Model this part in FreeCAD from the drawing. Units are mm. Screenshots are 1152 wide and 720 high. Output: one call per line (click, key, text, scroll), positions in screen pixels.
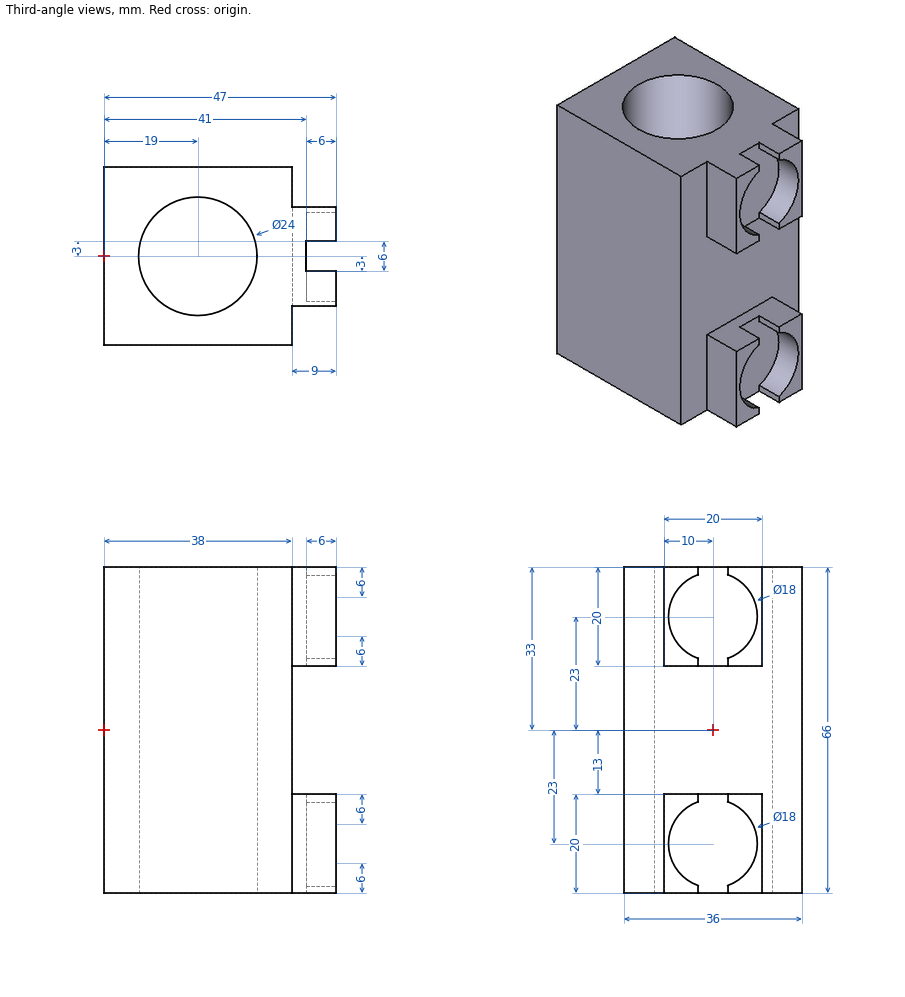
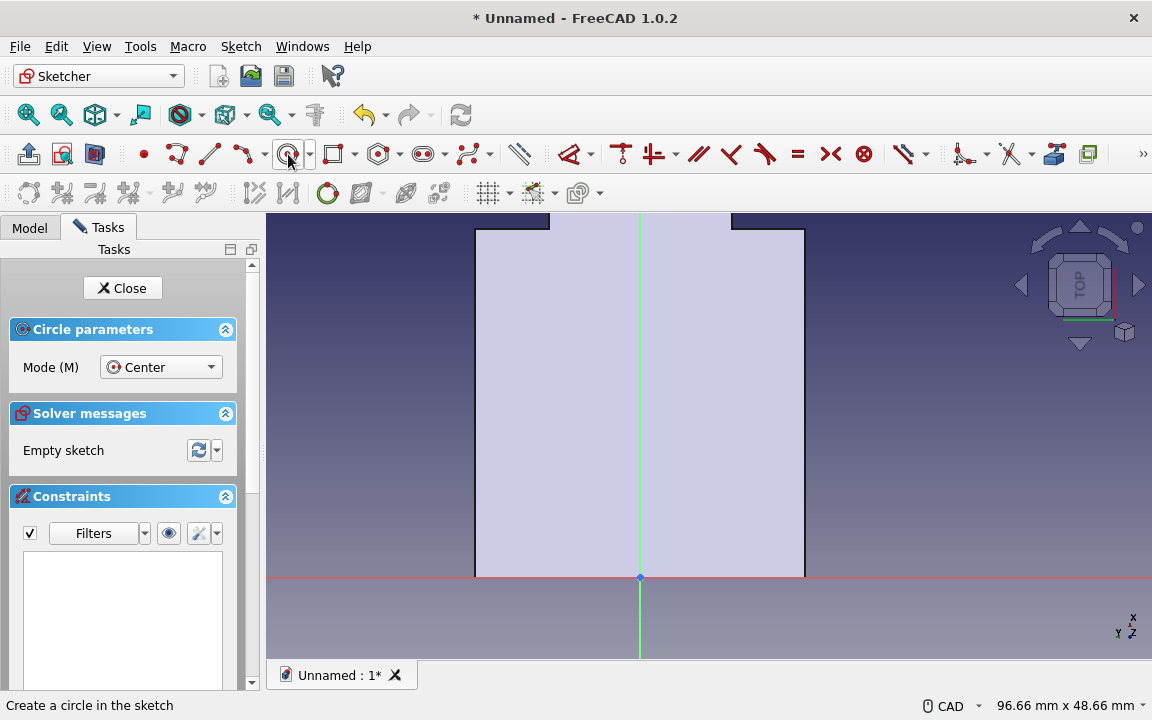
click(640, 404)
click(718, 326)
key(Escape)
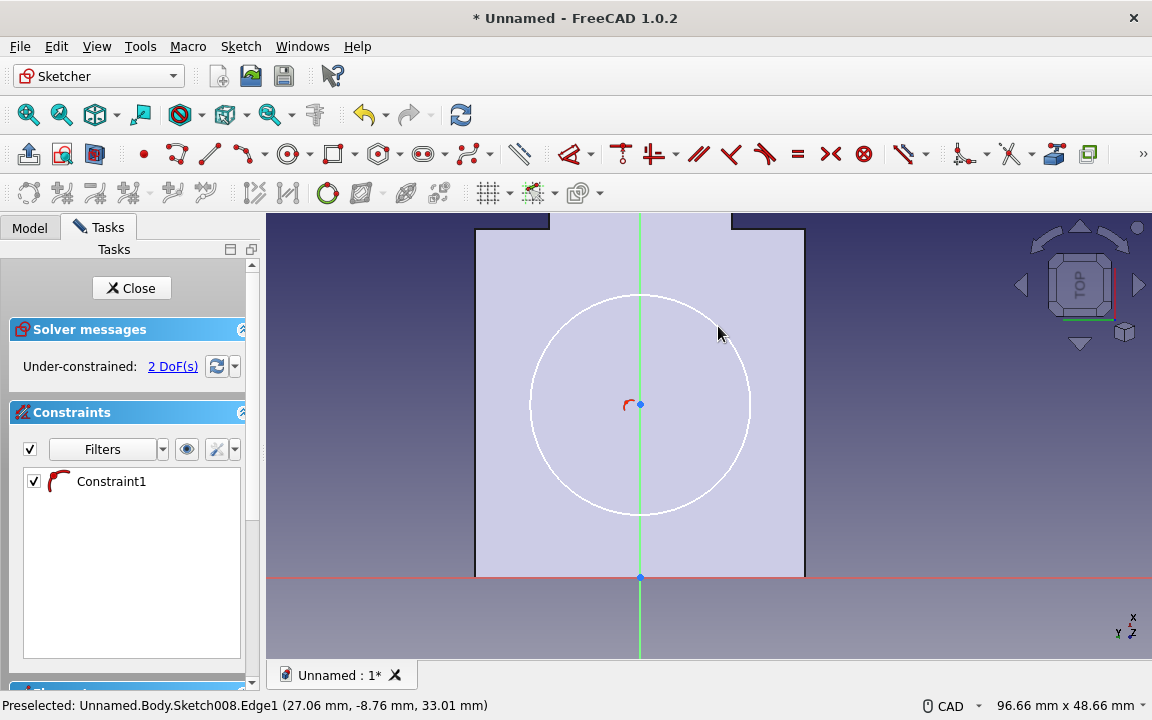
click(568, 154)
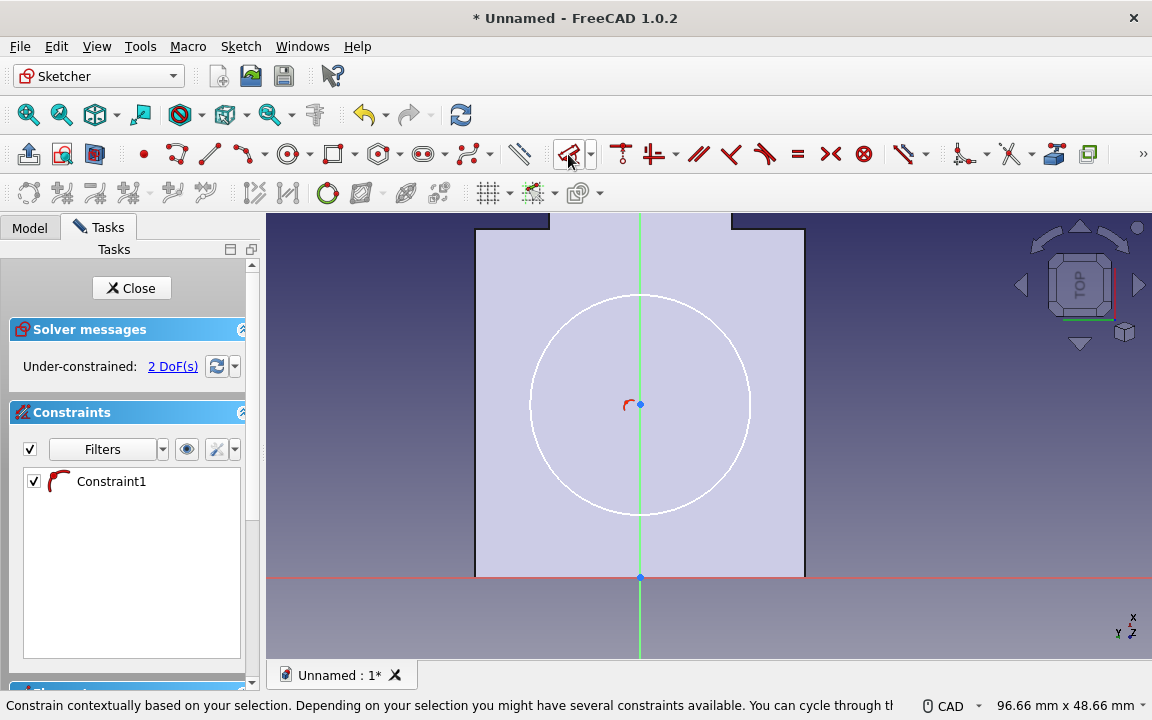
click(718, 327)
click(741, 304)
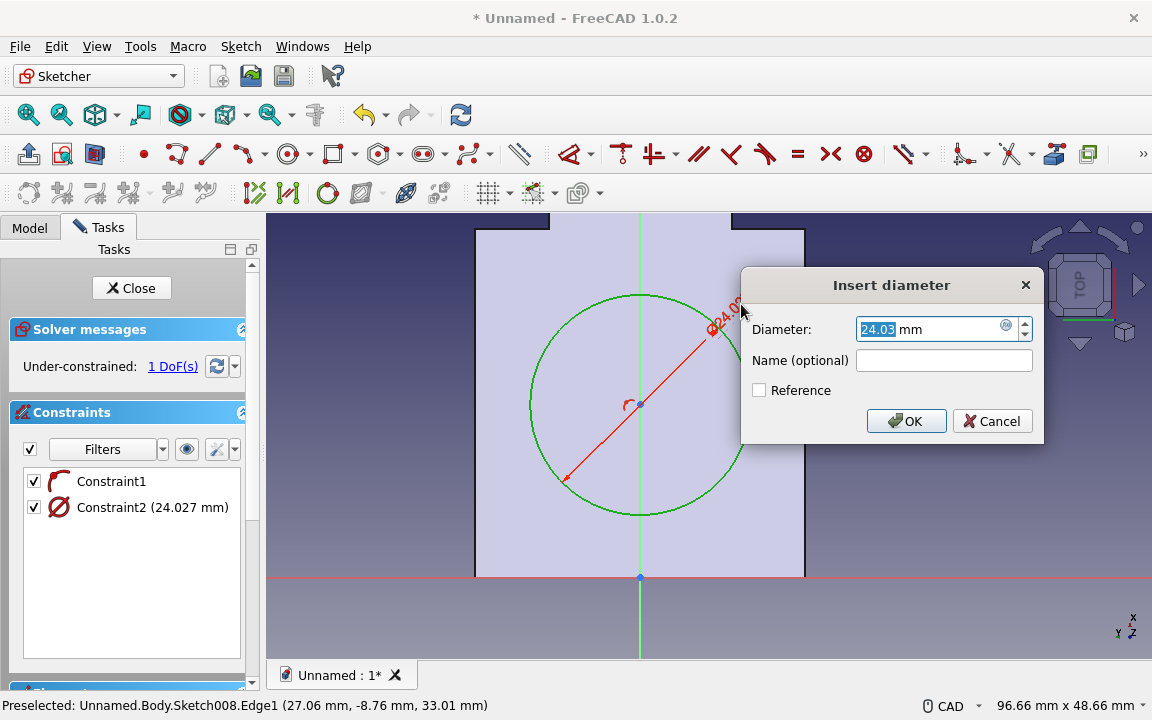
text(24)
key(Return)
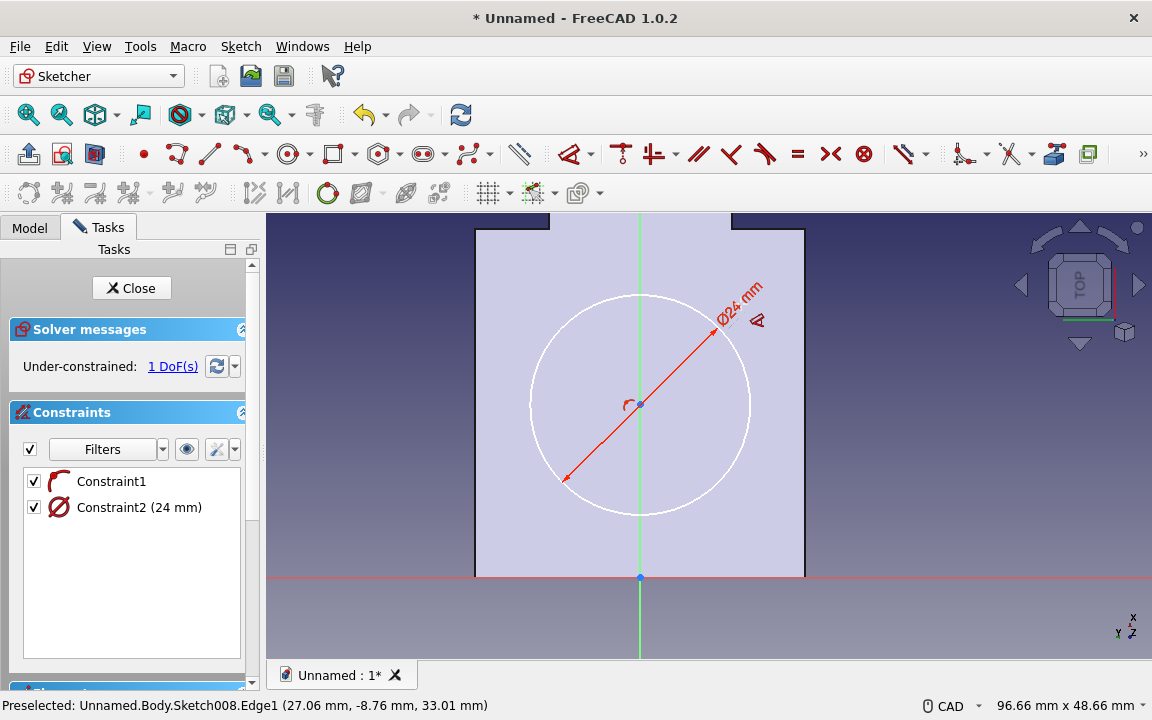
click(640, 405)
click(674, 491)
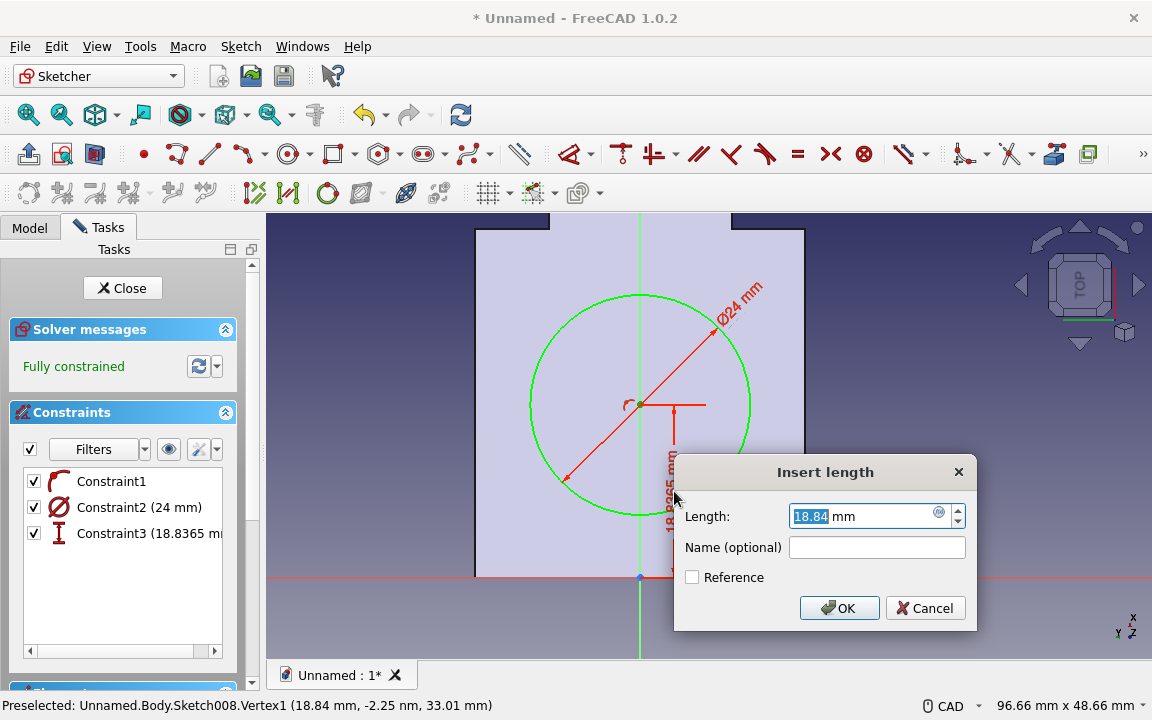
text(19)
key(Return)
key(Escape)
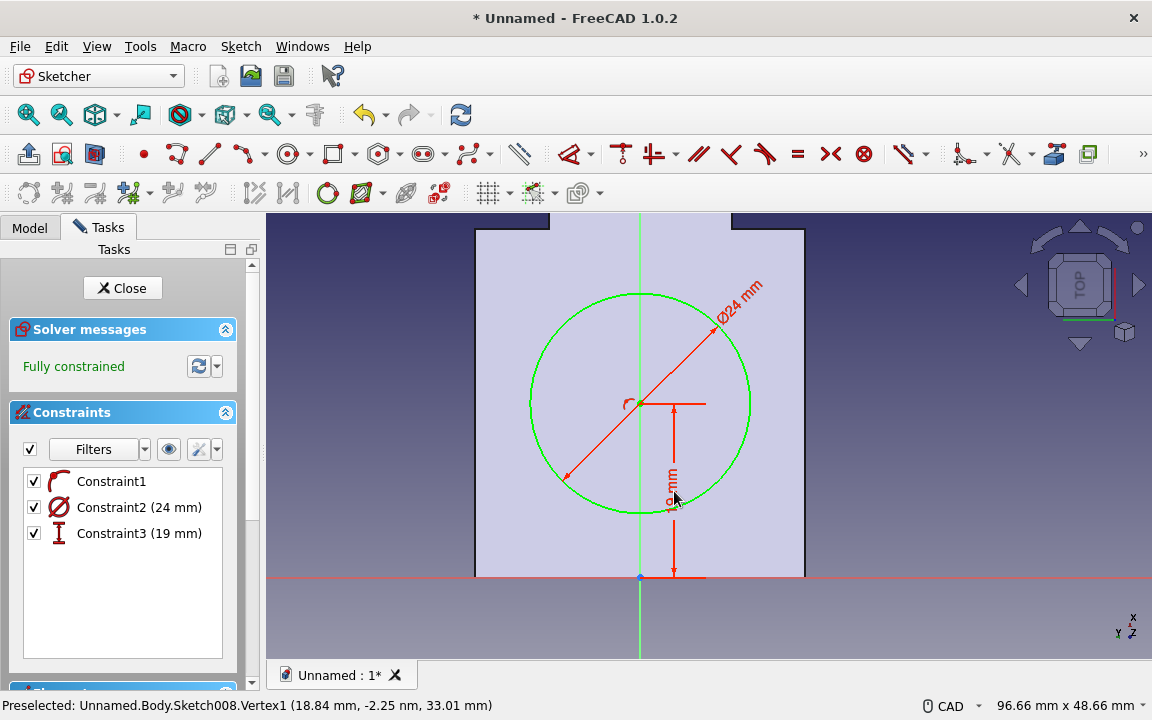
click(123, 288)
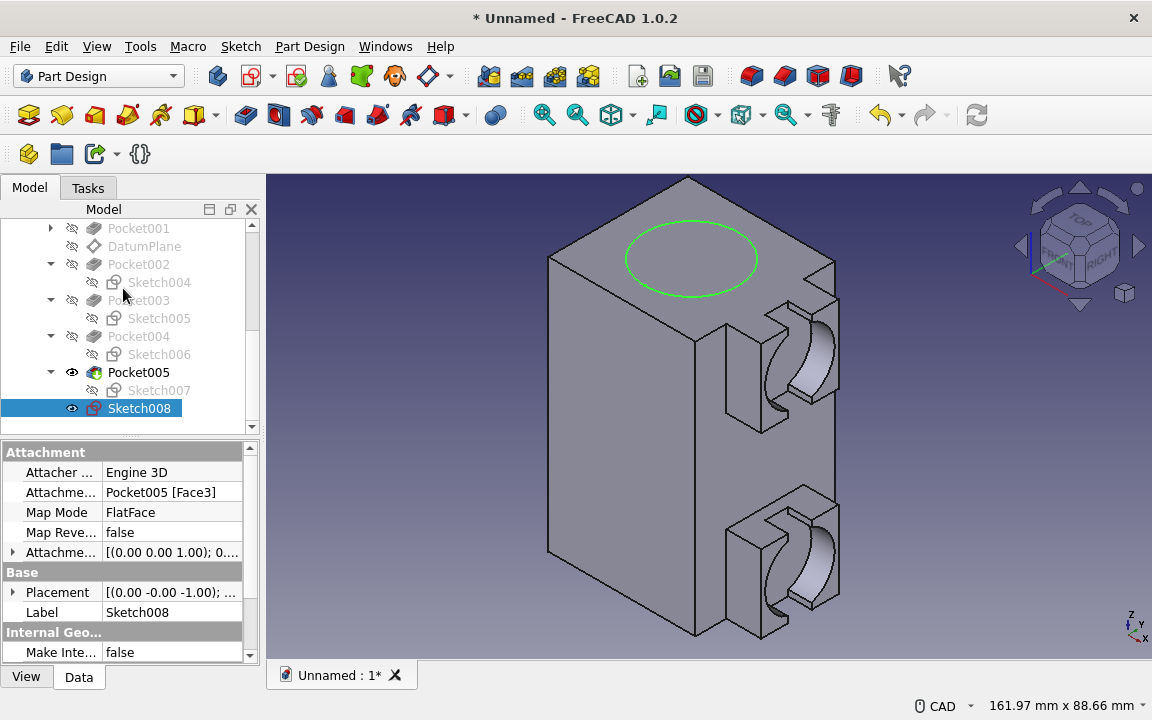
click(246, 116)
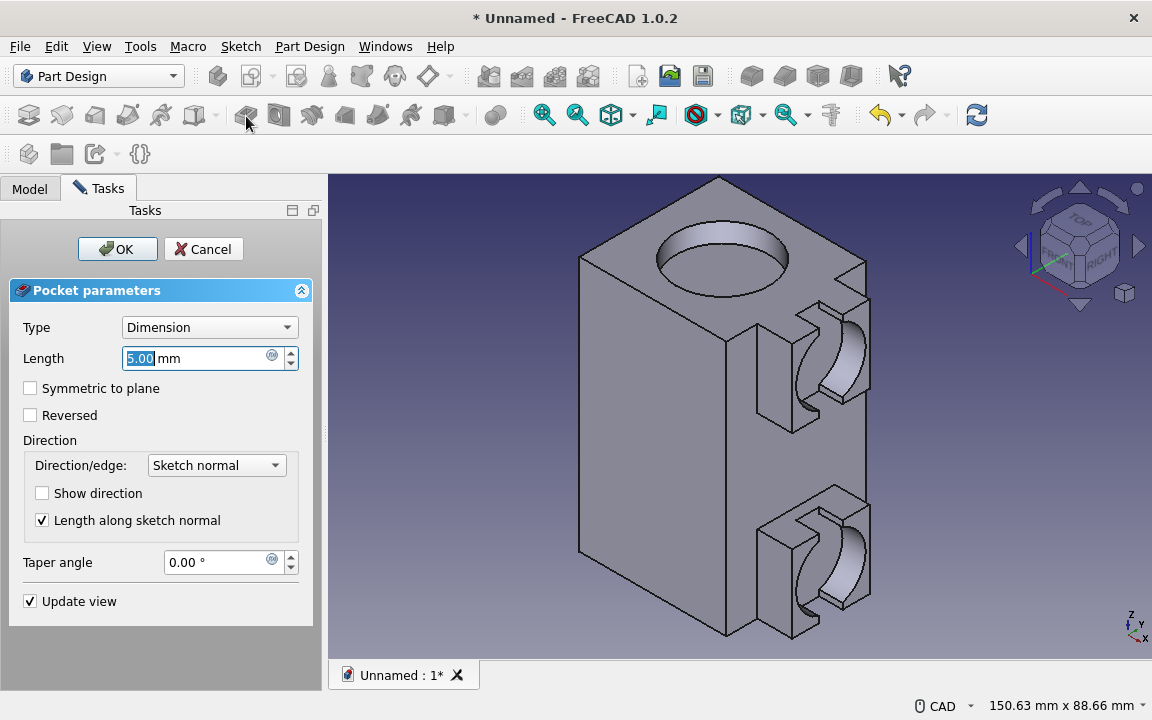
click(210, 328)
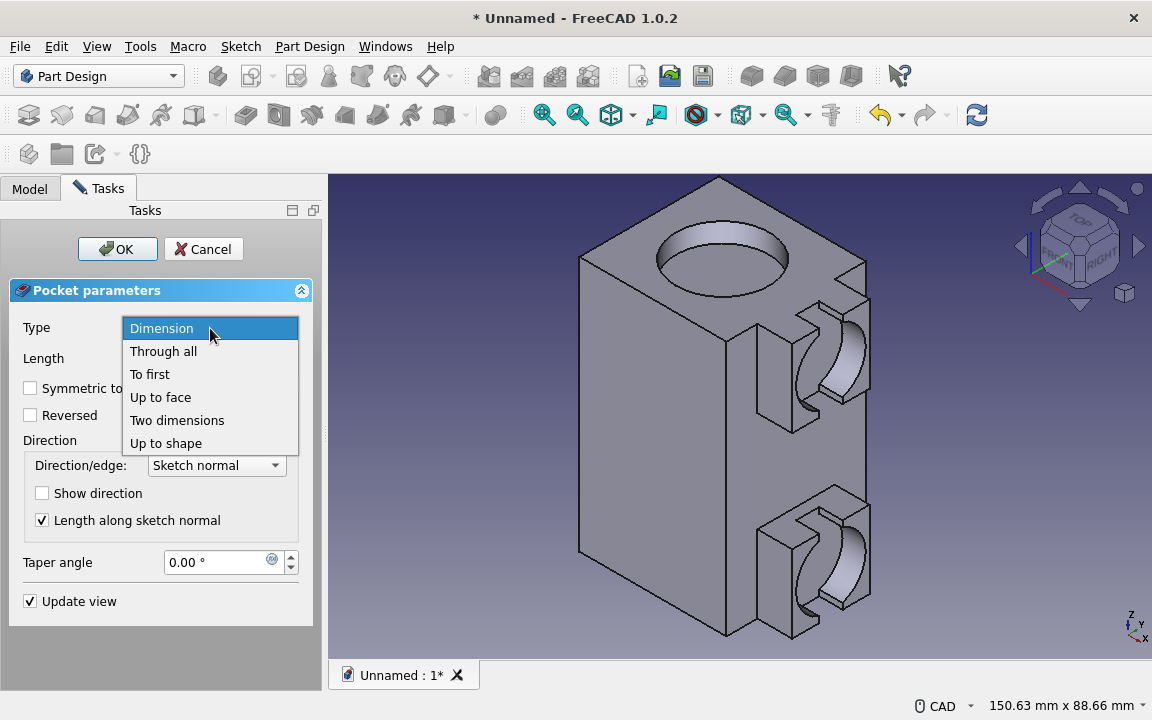
click(208, 352)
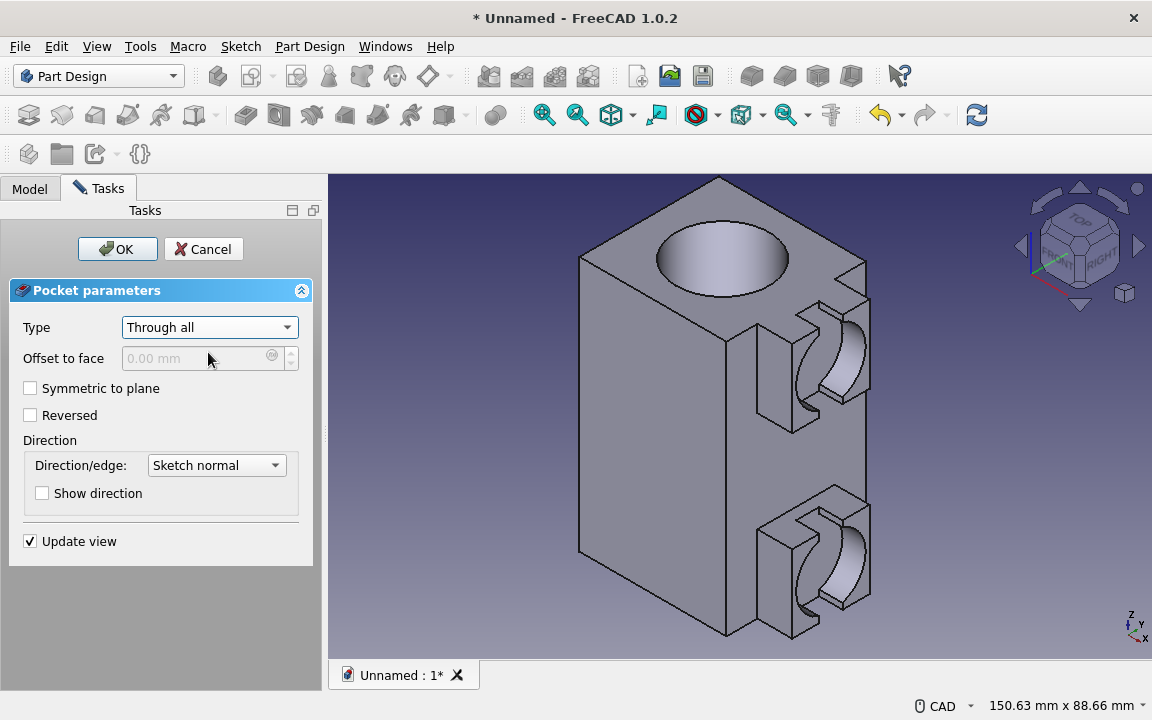
click(118, 249)